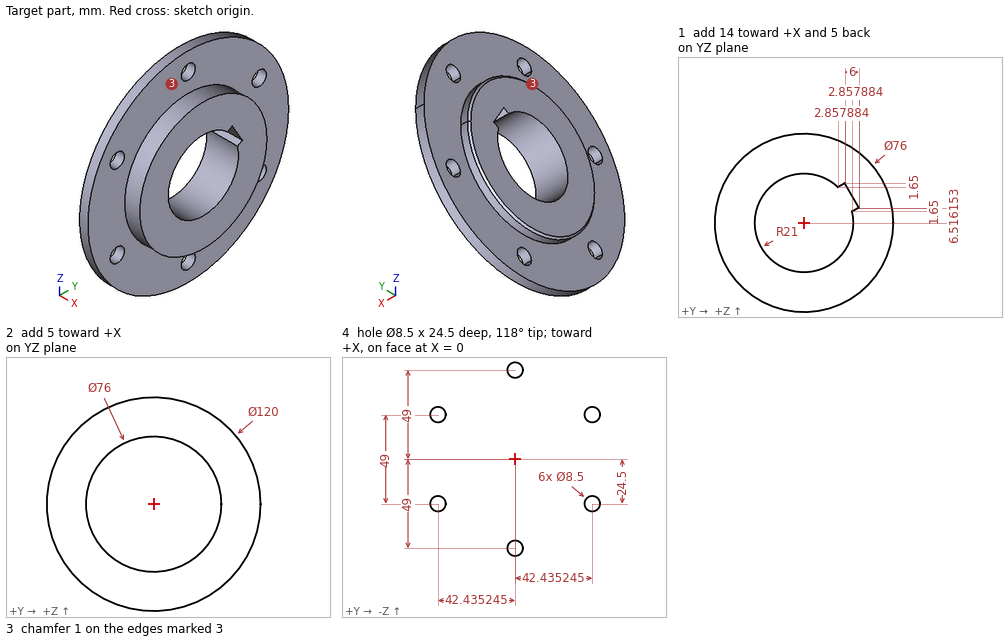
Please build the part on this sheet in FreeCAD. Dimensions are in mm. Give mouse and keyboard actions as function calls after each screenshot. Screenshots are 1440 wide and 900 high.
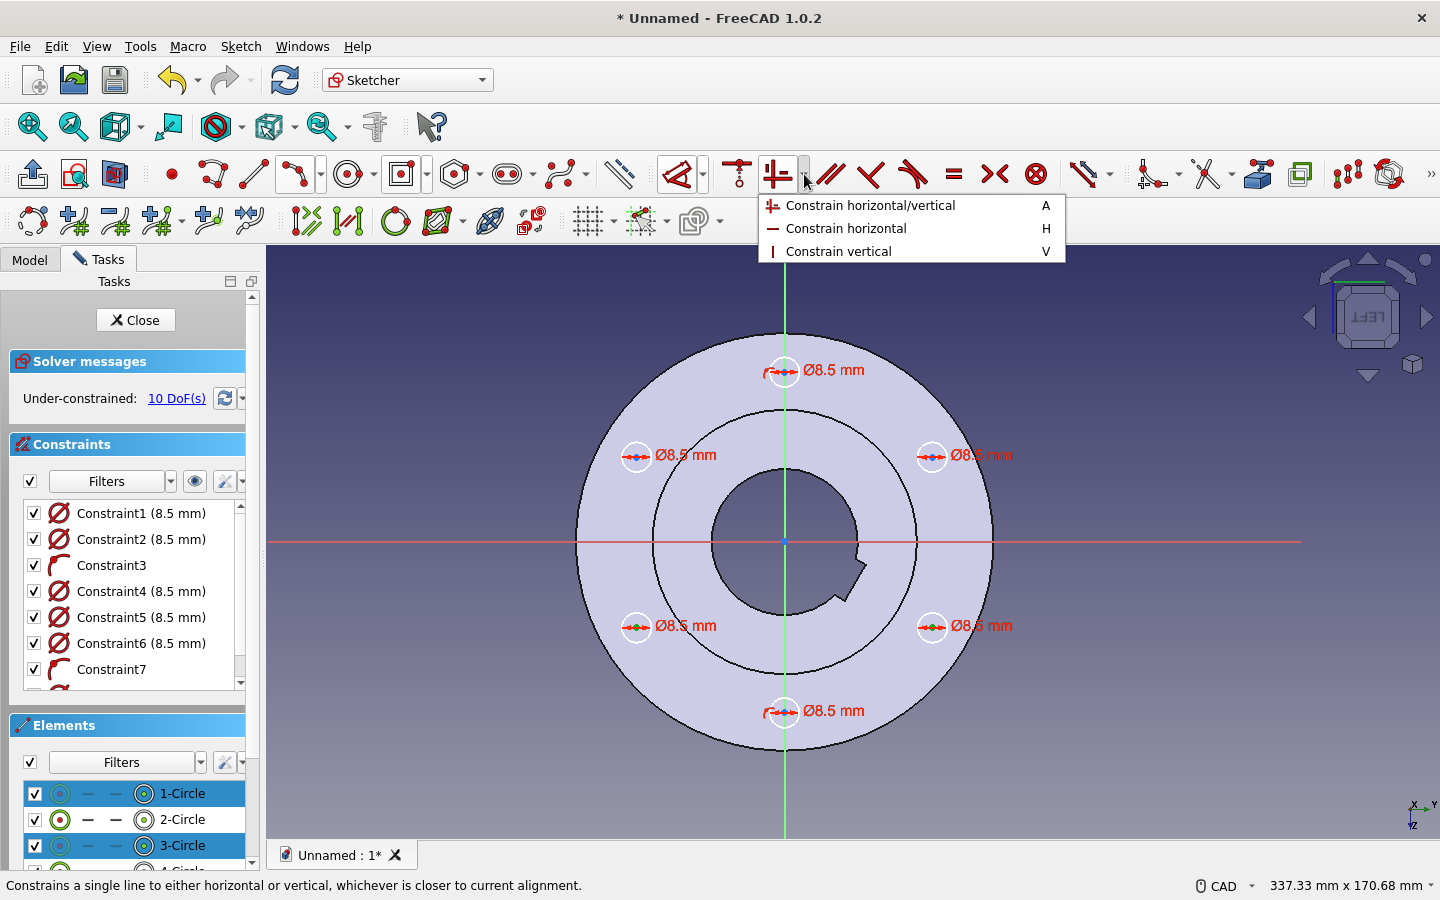
click(912, 228)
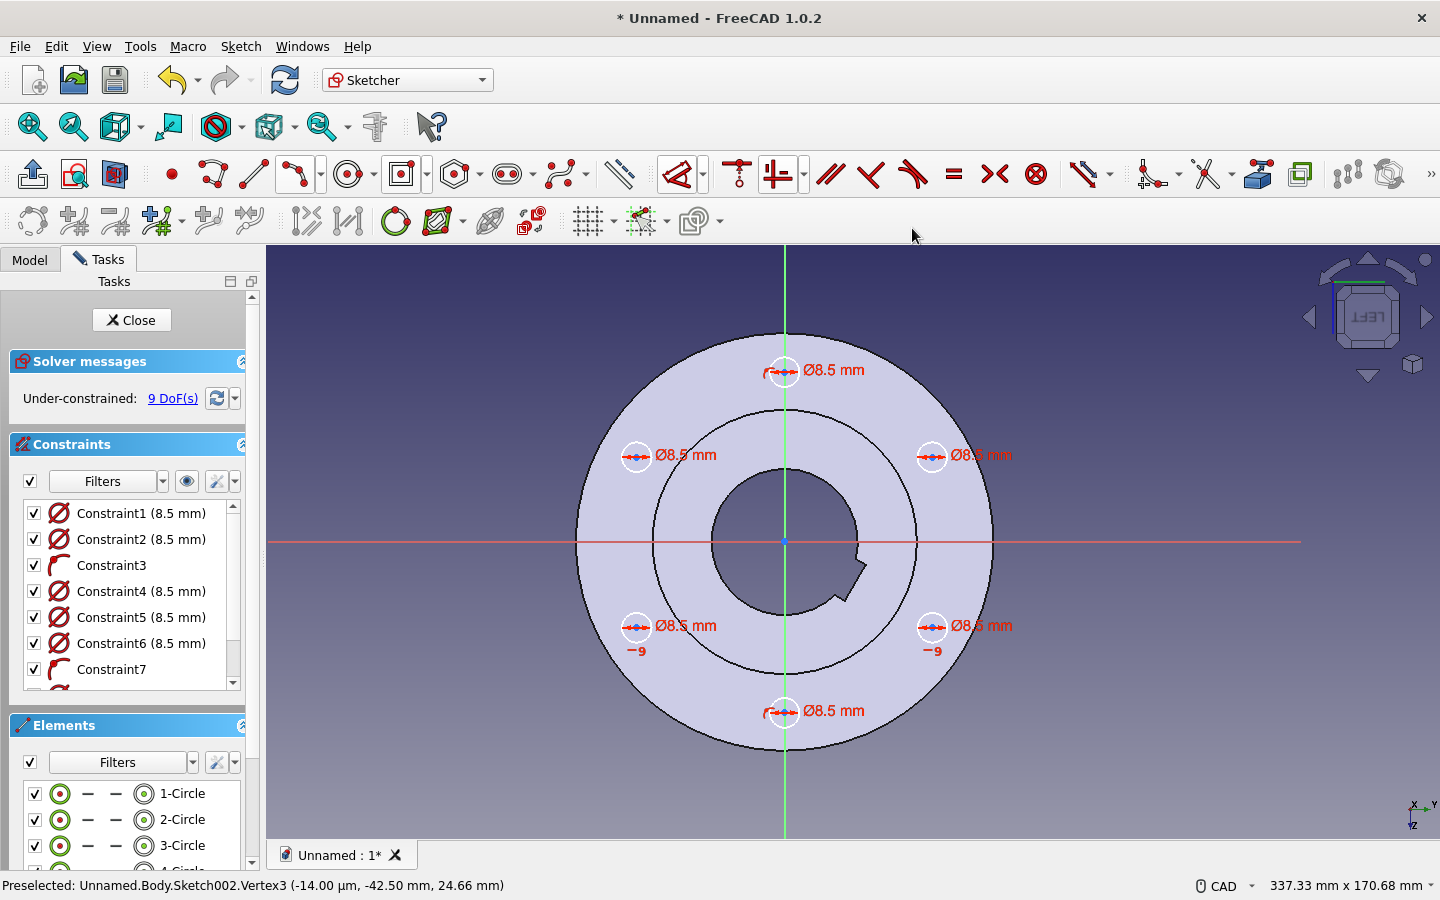
click(637, 628)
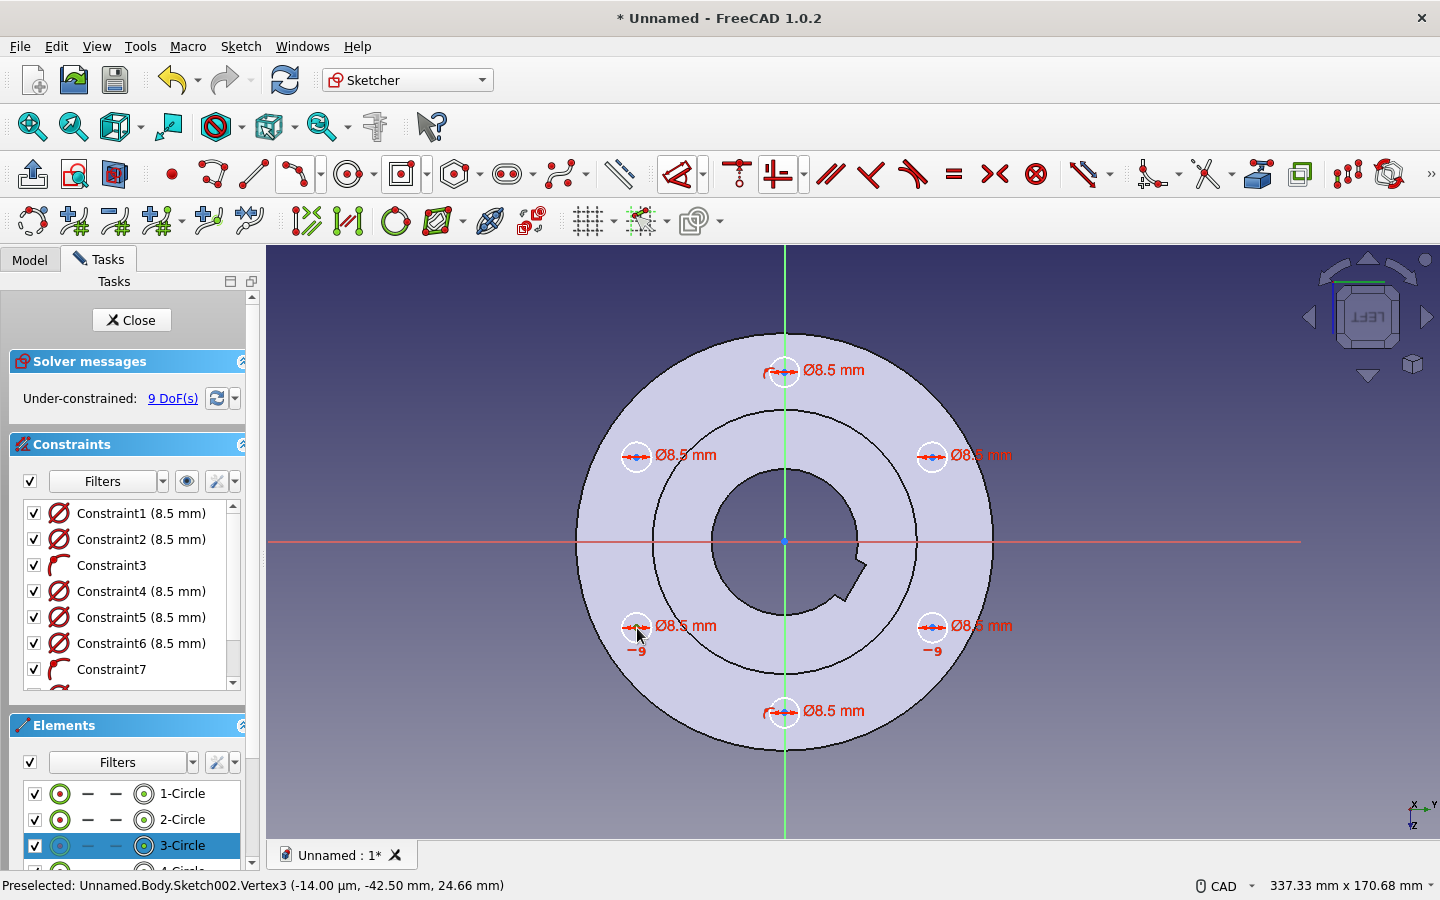
click(637, 457)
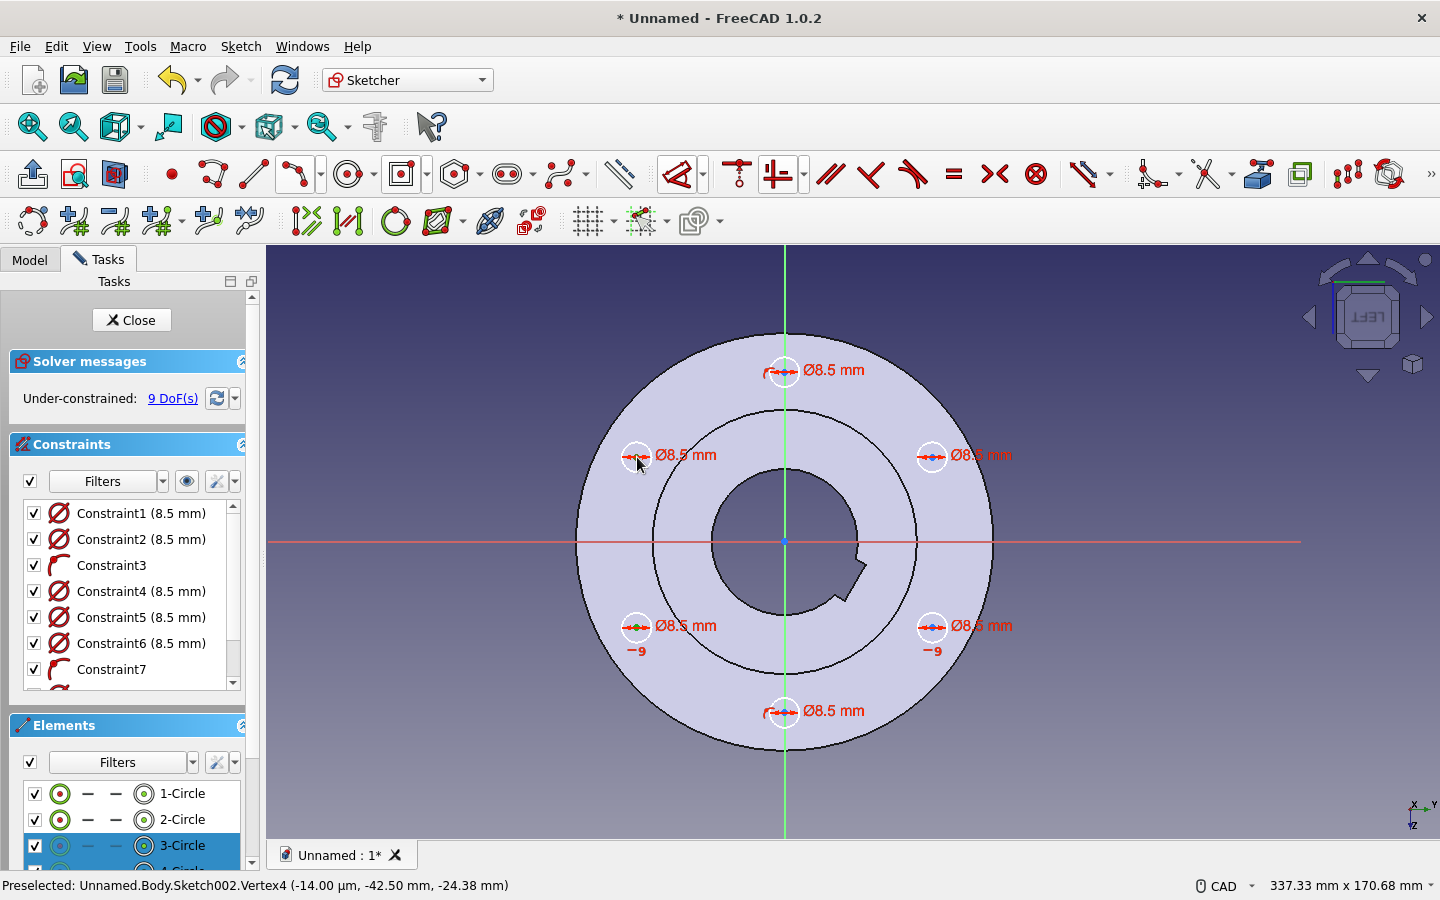
key(v)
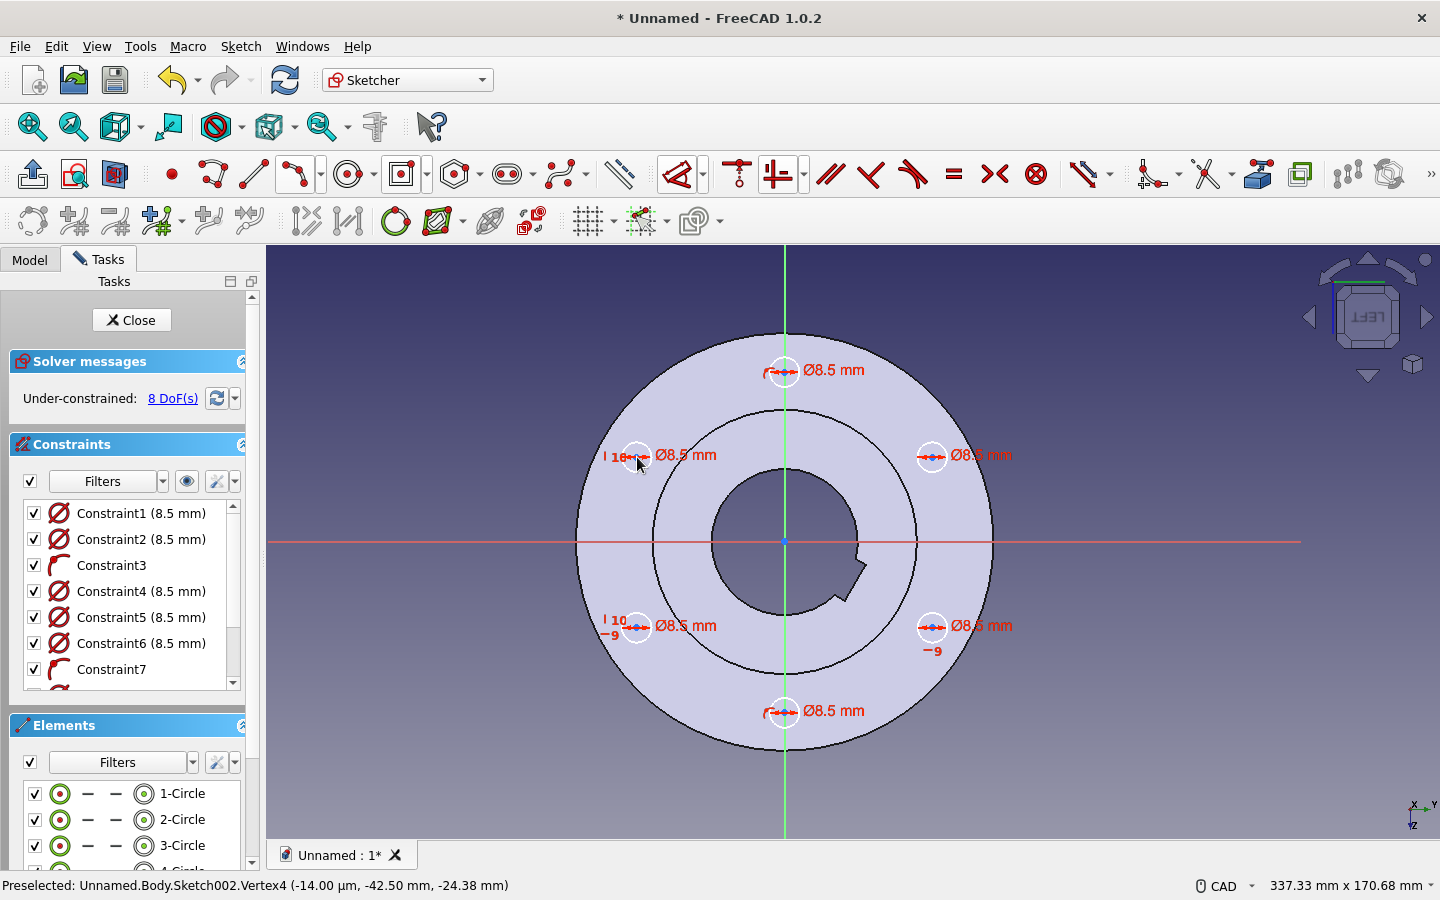
click(933, 628)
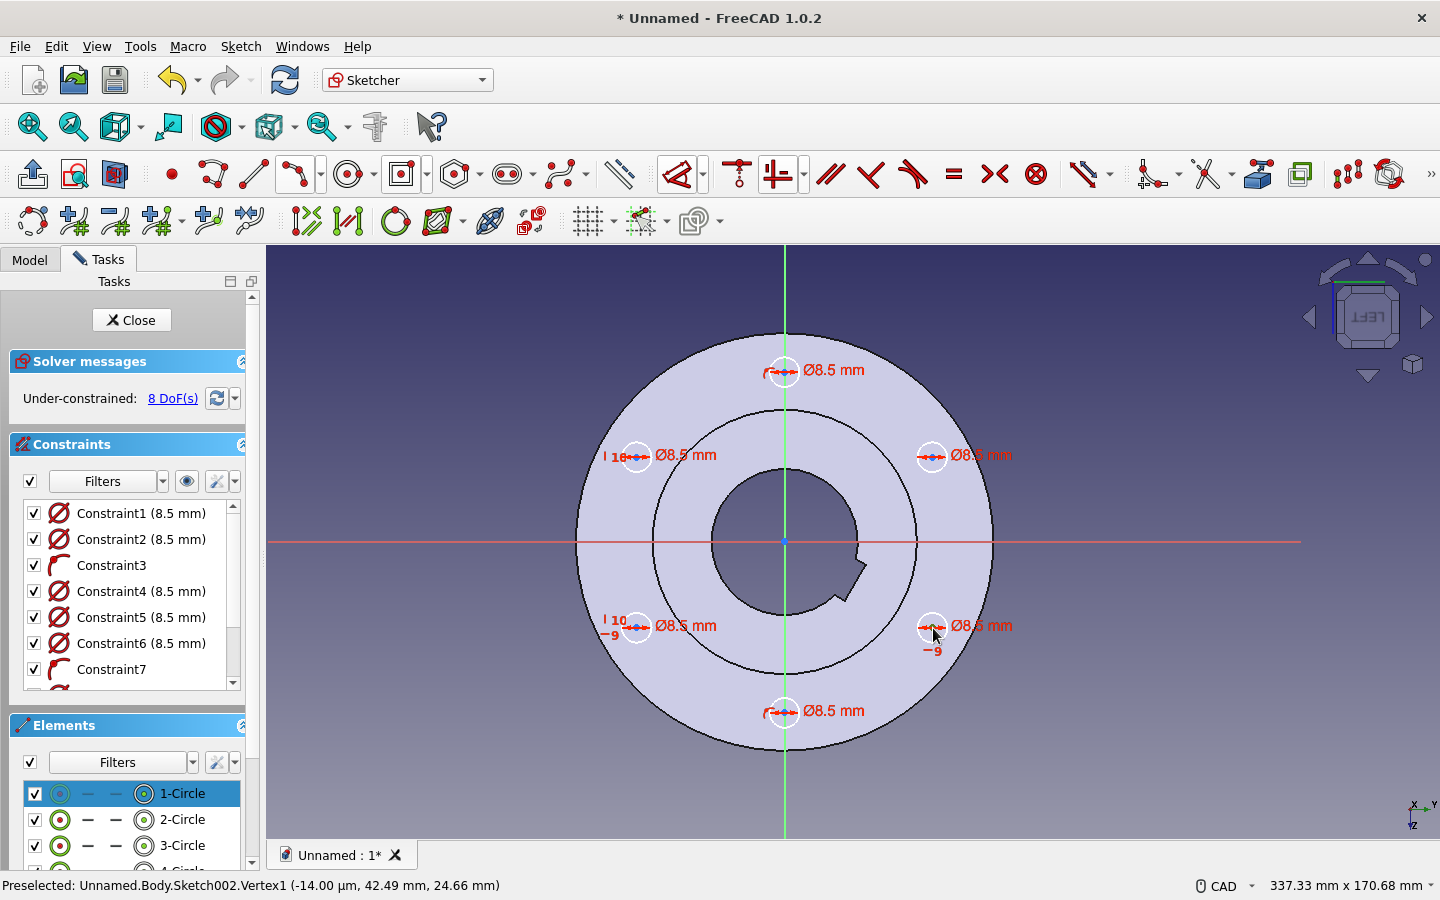
click(932, 457)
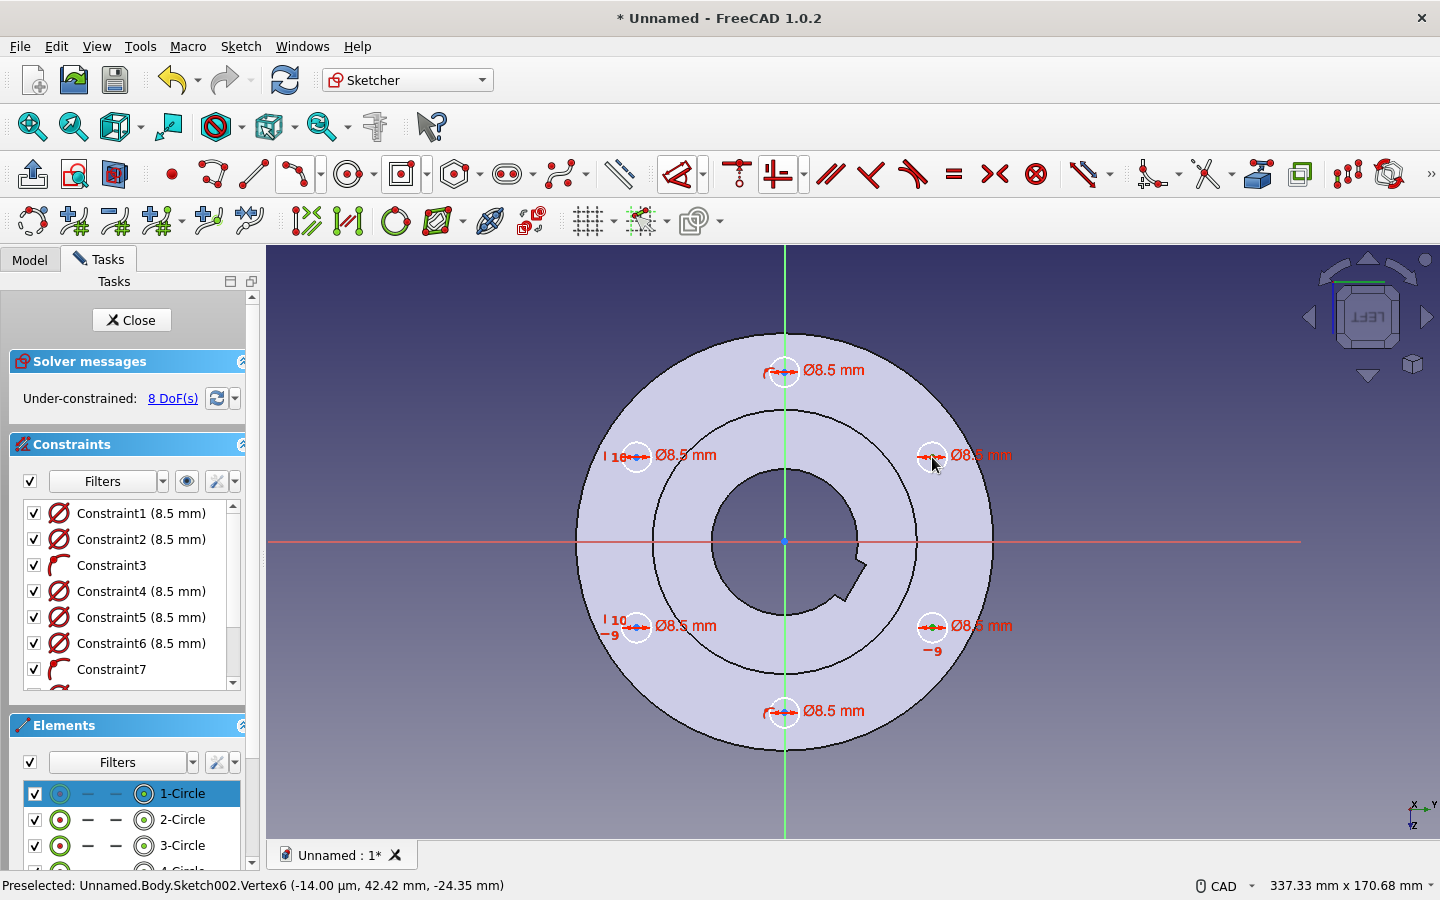
click(804, 174)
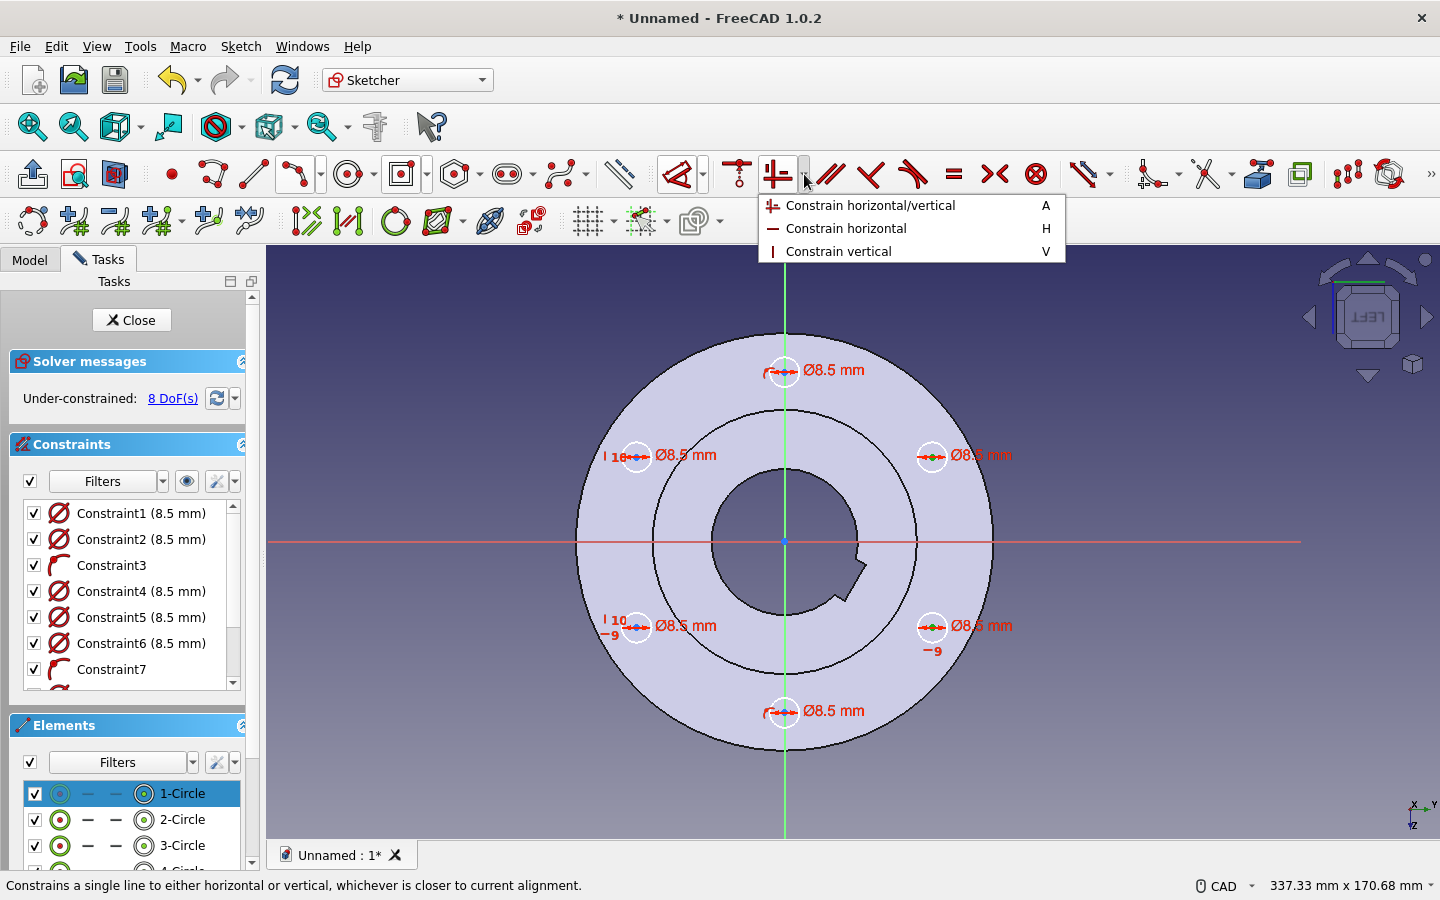
click(912, 252)